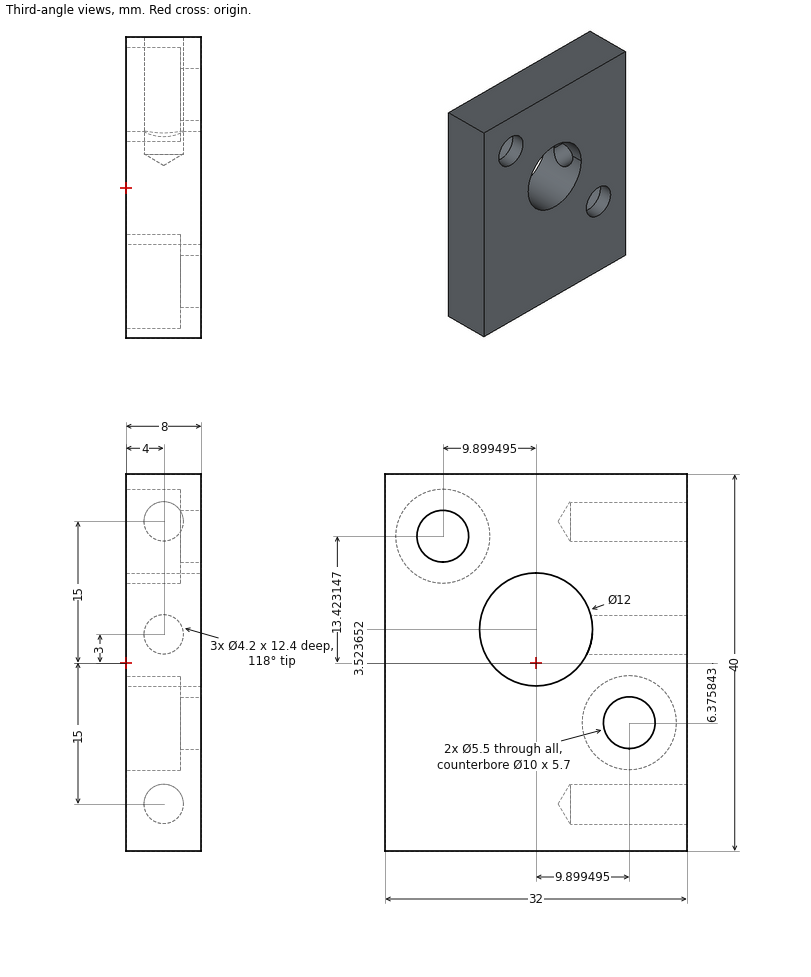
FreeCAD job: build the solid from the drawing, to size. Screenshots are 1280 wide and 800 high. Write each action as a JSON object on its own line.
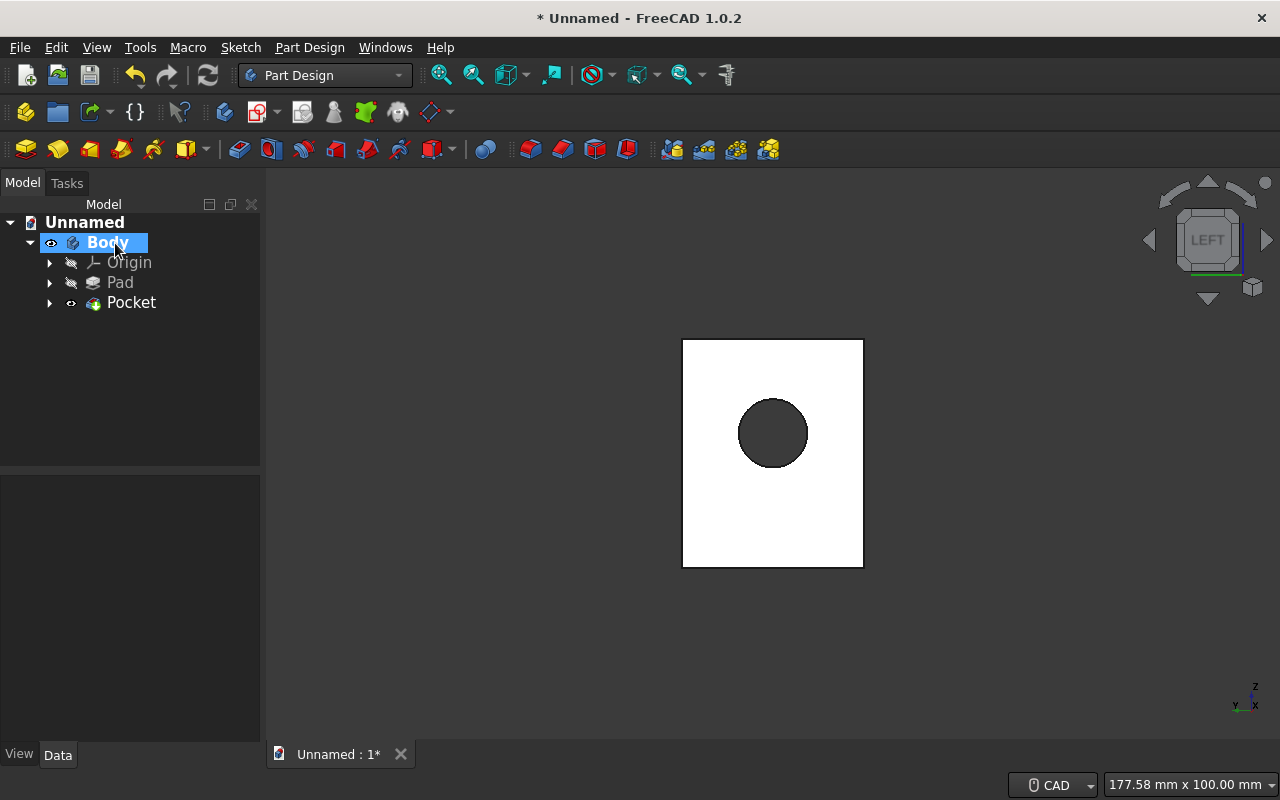
{"action": "key", "text": "v f"}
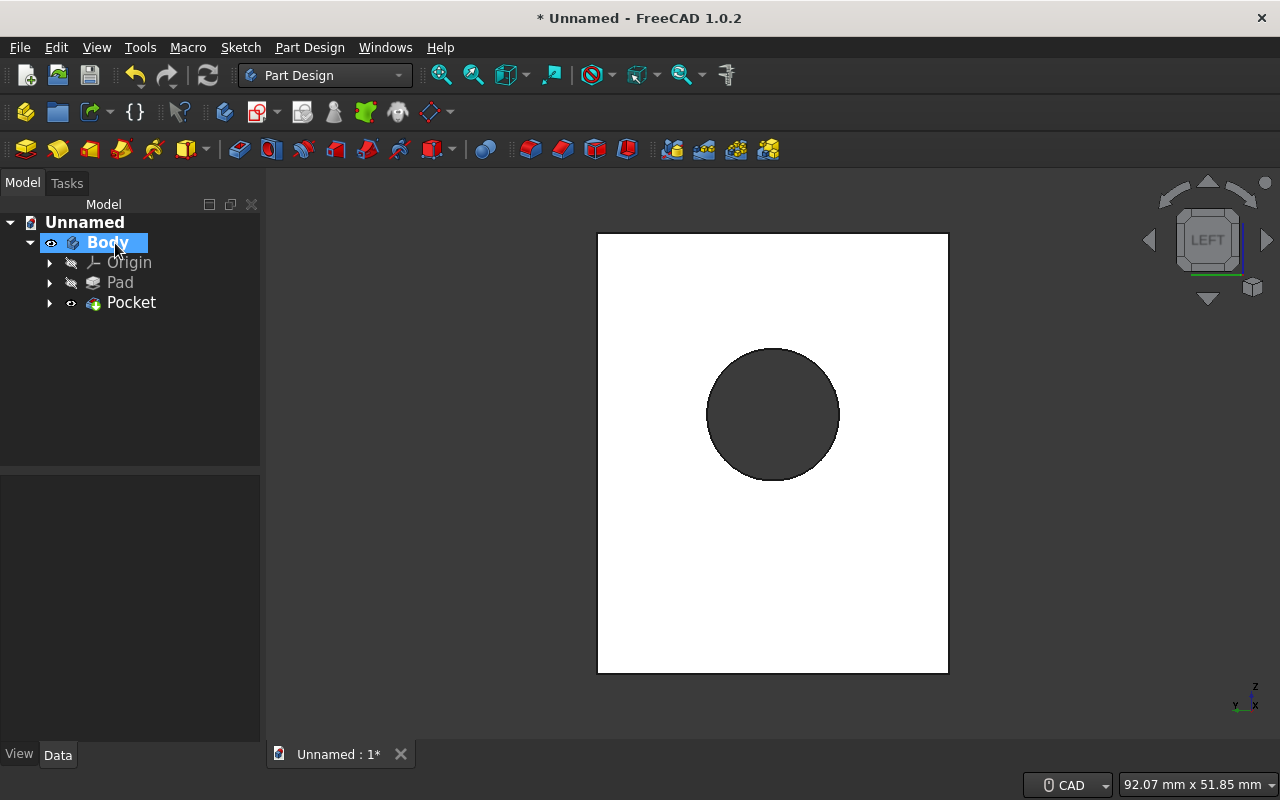
{"action": "left_click", "coordinate": [723, 578]}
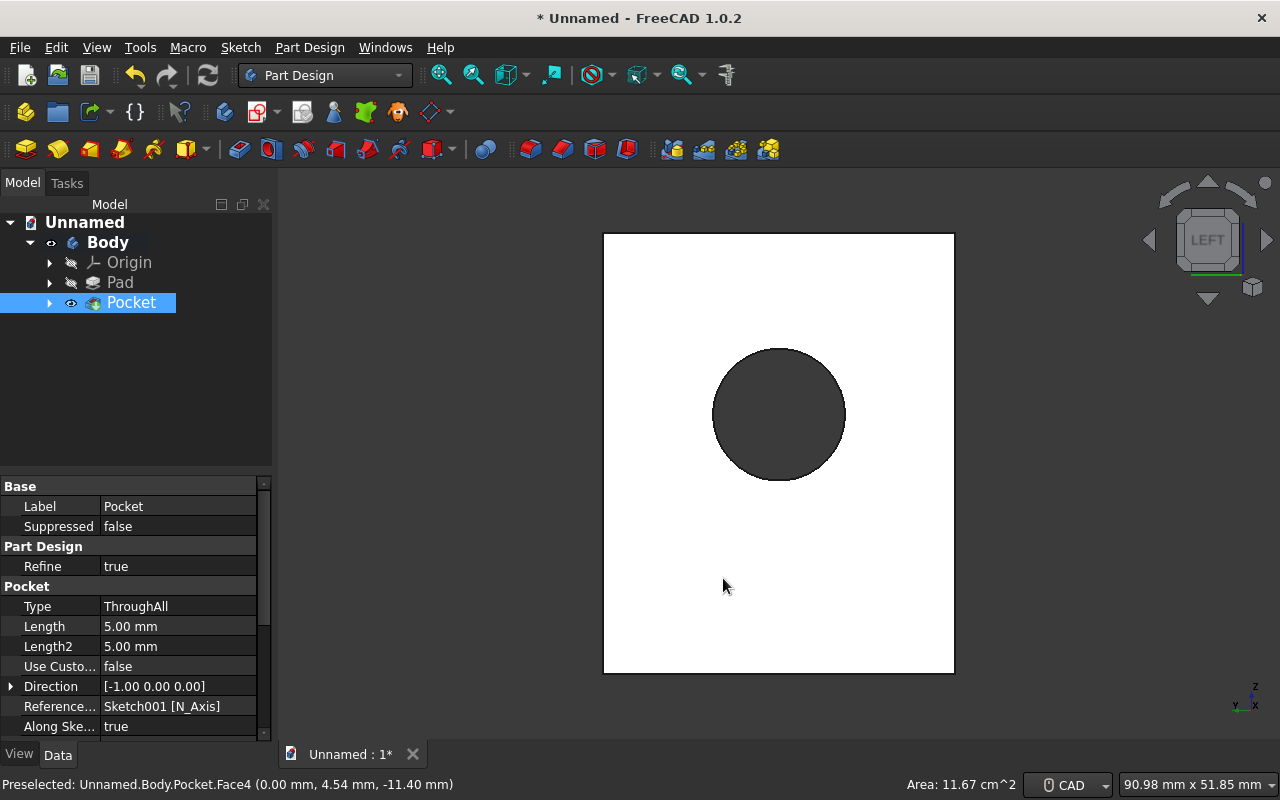
{"action": "left_click", "coordinate": [258, 112]}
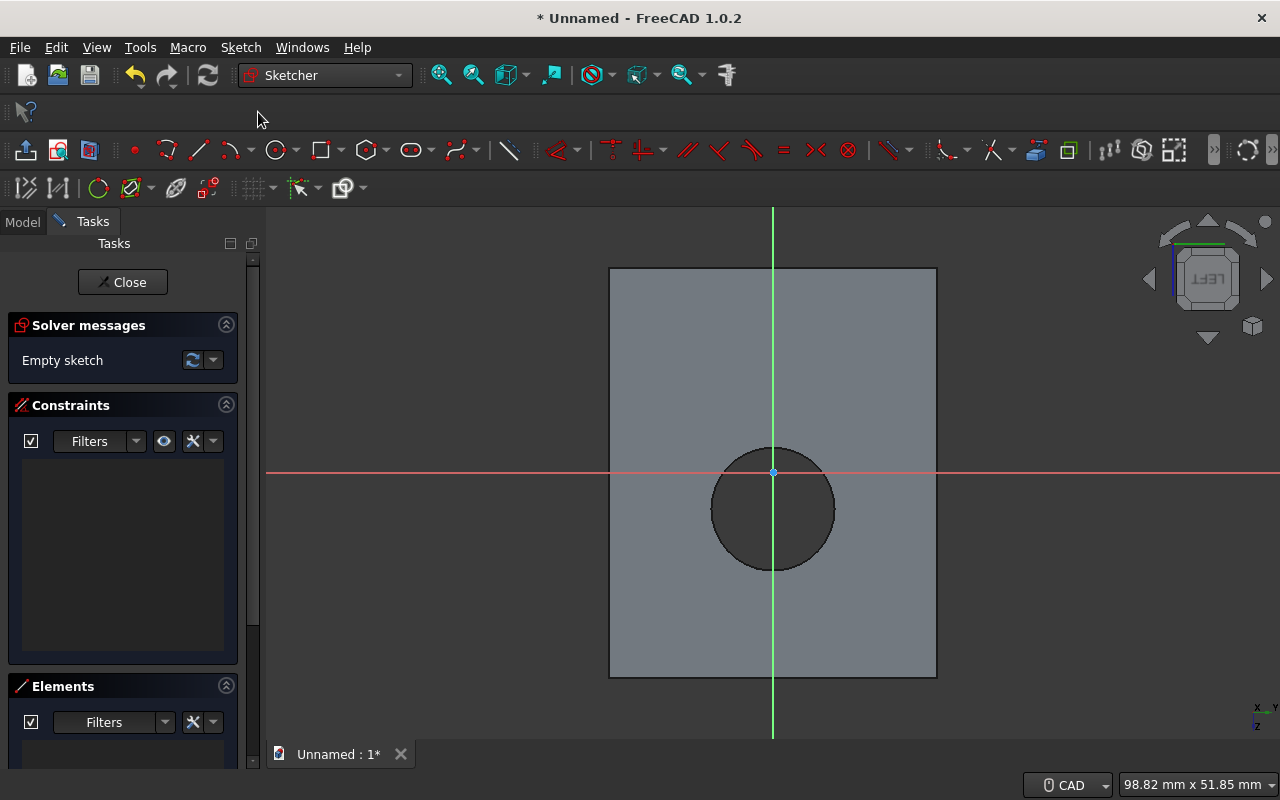
{"action": "key", "text": "g c"}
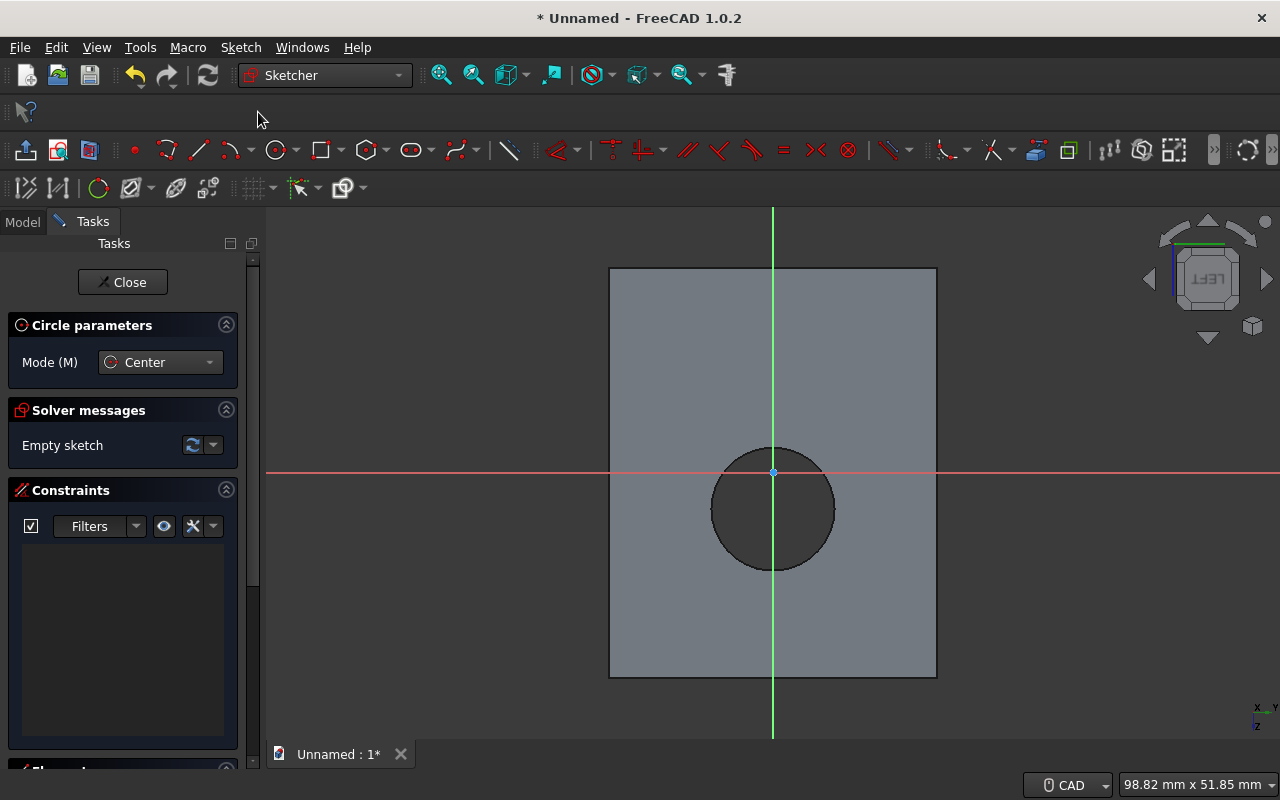
{"action": "left_click", "coordinate": [875, 408]}
{"action": "mouse_move", "coordinate": [895, 388]}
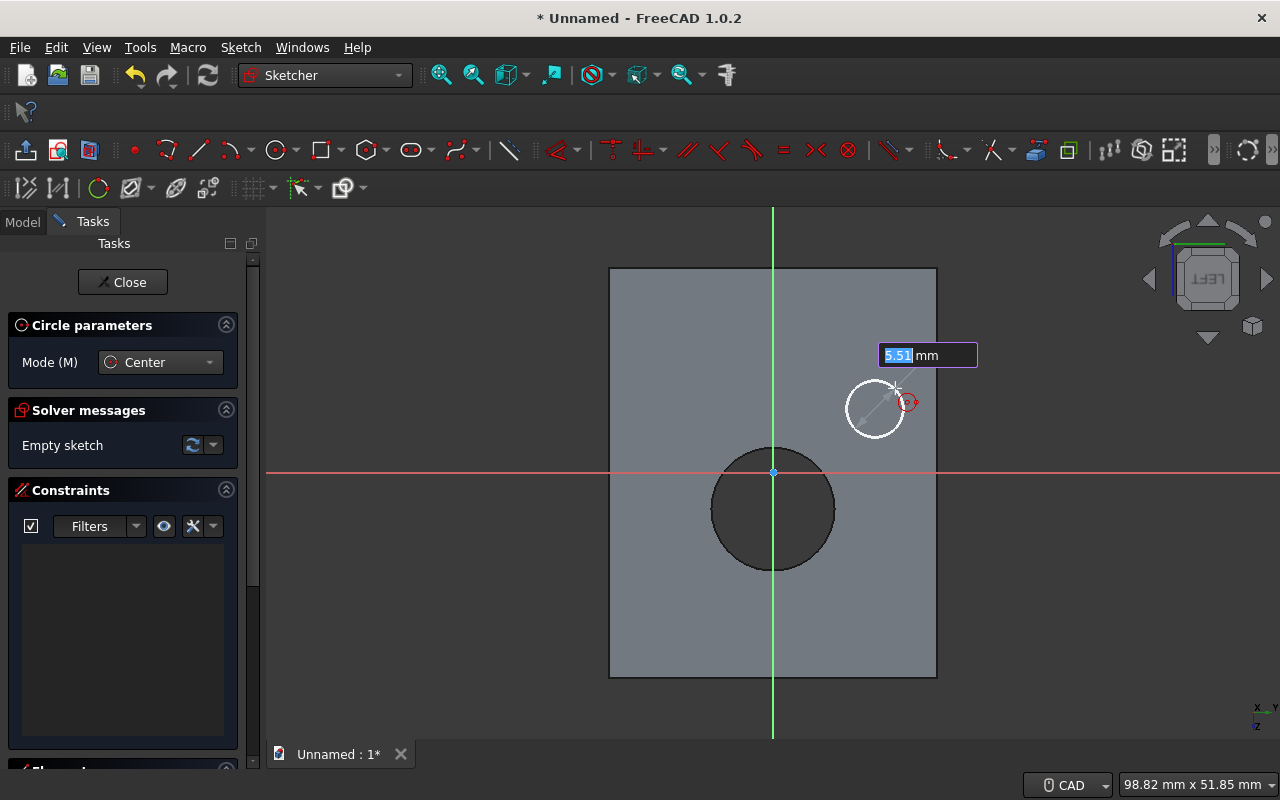
{"action": "type", "text": "5.5"}
{"action": "key", "text": "Return"}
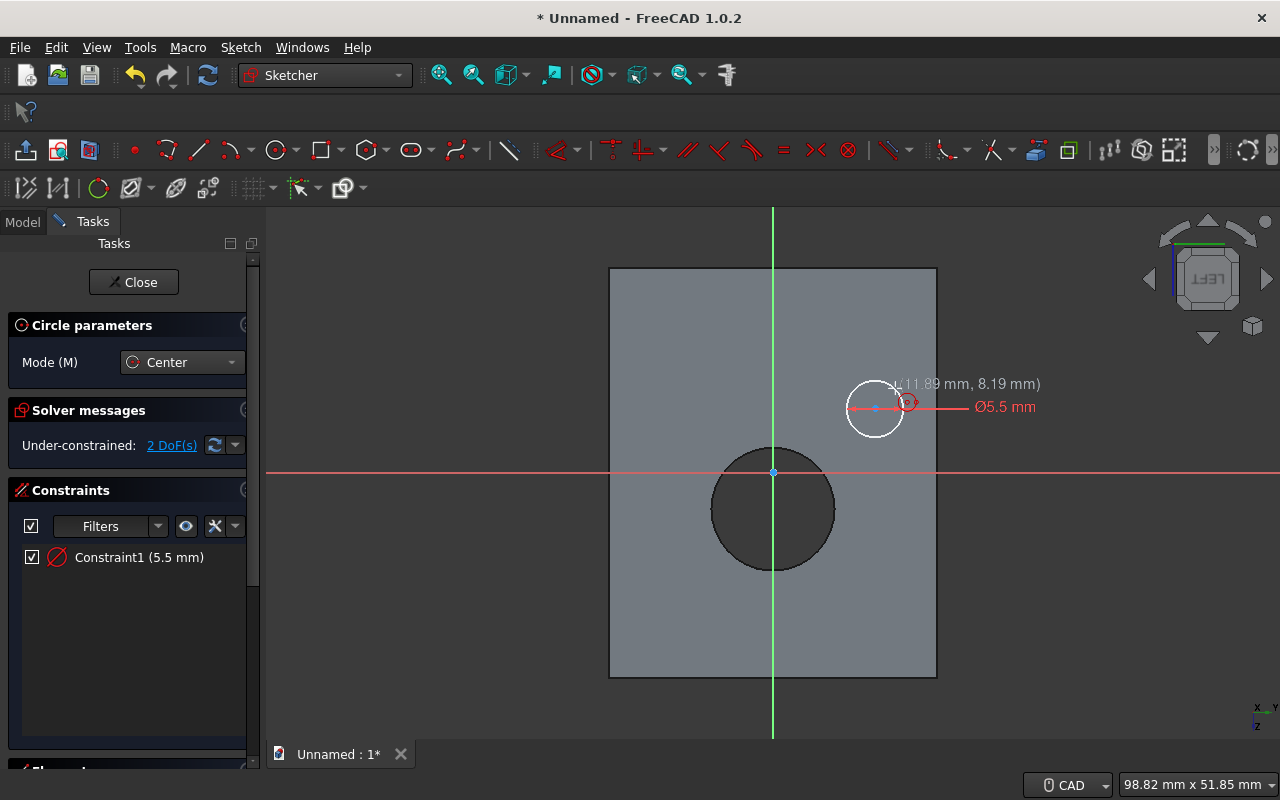
{"action": "left_click", "coordinate": [671, 611]}
{"action": "mouse_move", "coordinate": [691, 591]}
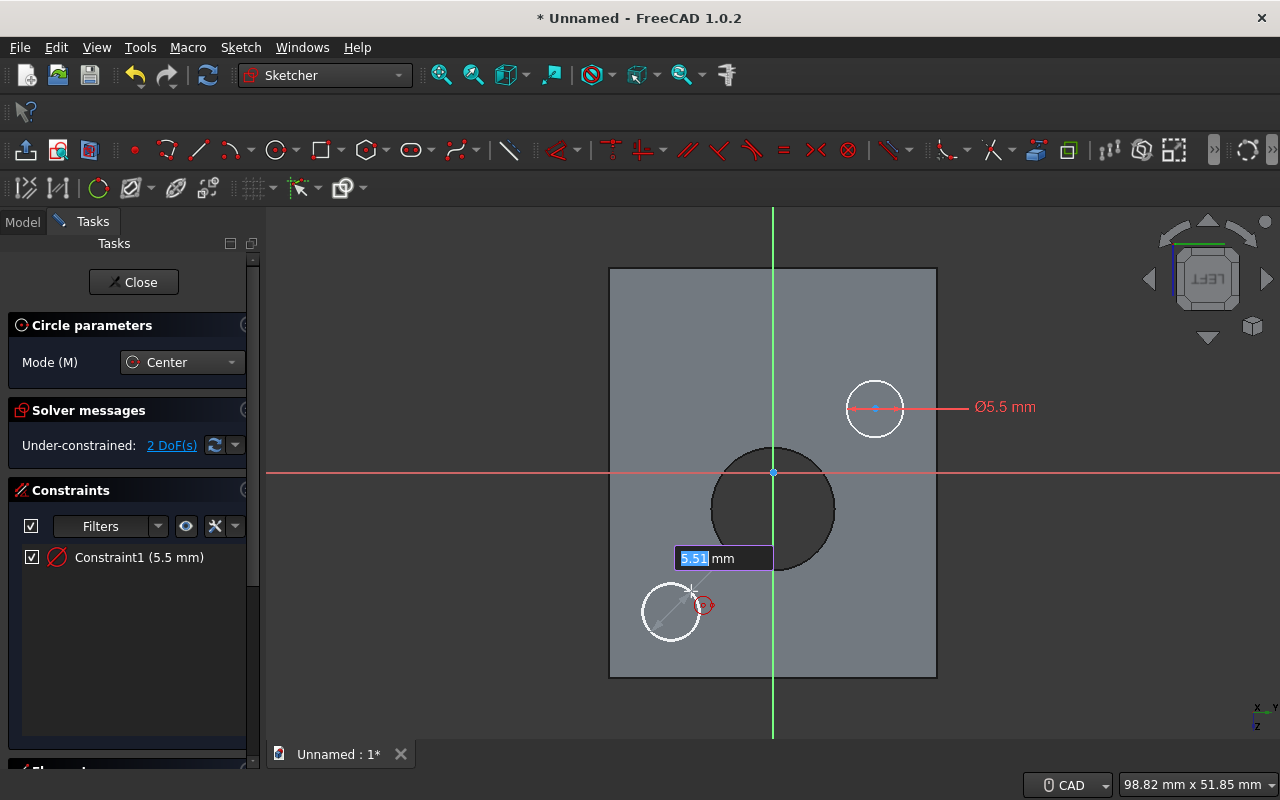
{"action": "type", "text": "5.5"}
{"action": "key", "text": "Return"}
{"action": "key", "text": "Escape"}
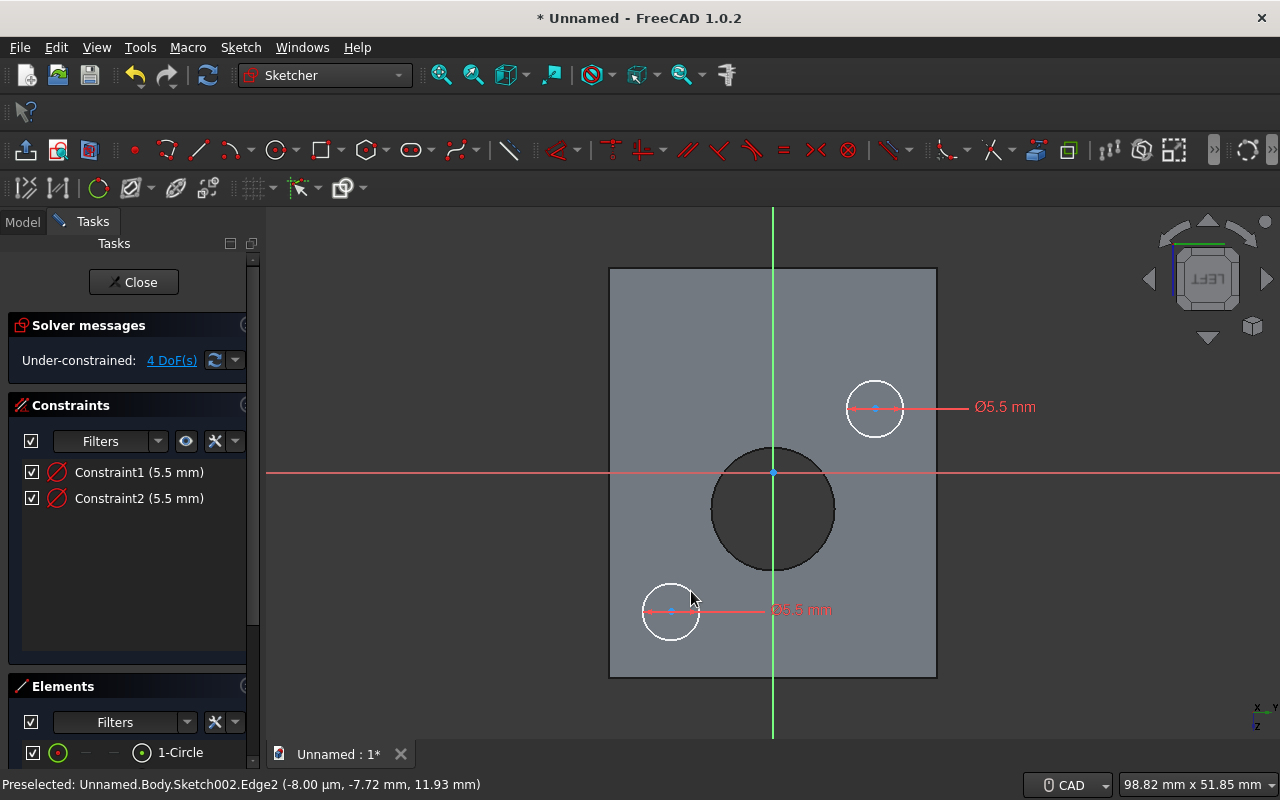
{"action": "key", "text": "d"}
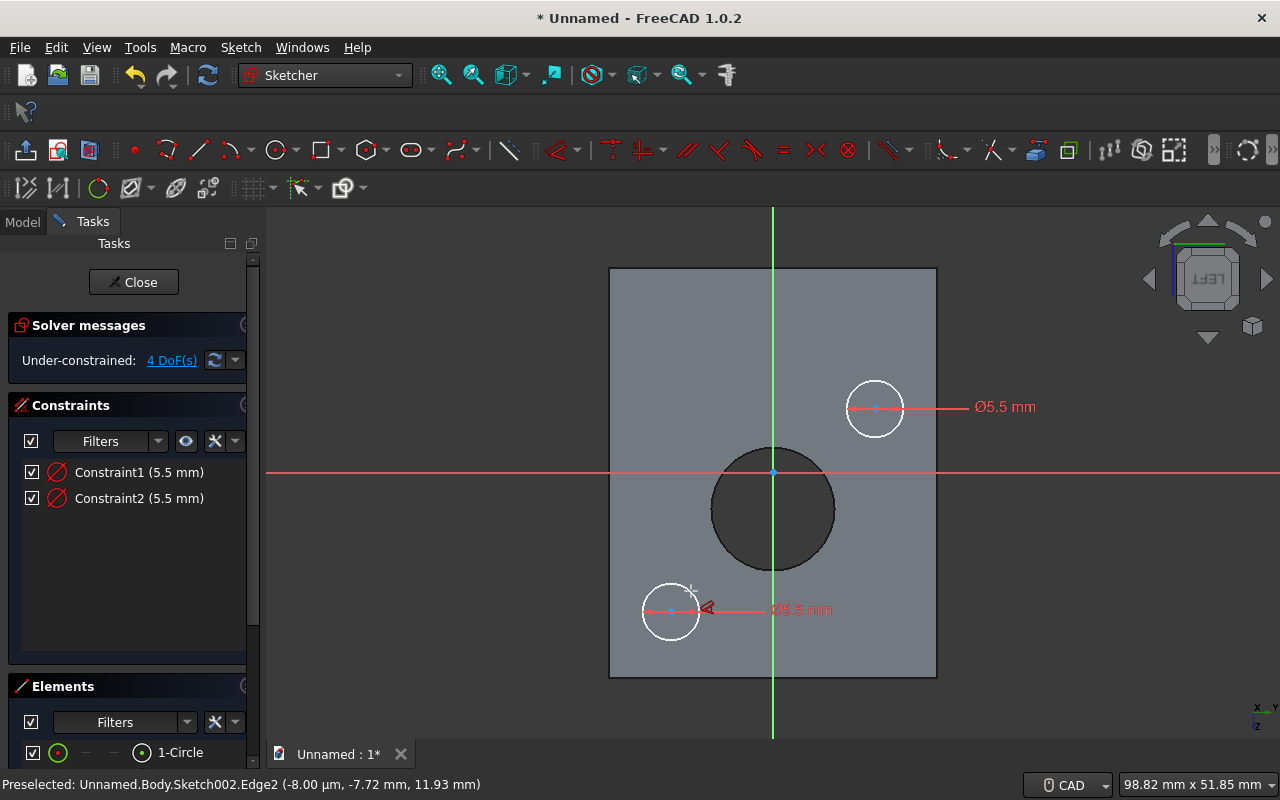
{"action": "left_click", "coordinate": [875, 409]}
{"action": "left_click", "coordinate": [824, 375]}